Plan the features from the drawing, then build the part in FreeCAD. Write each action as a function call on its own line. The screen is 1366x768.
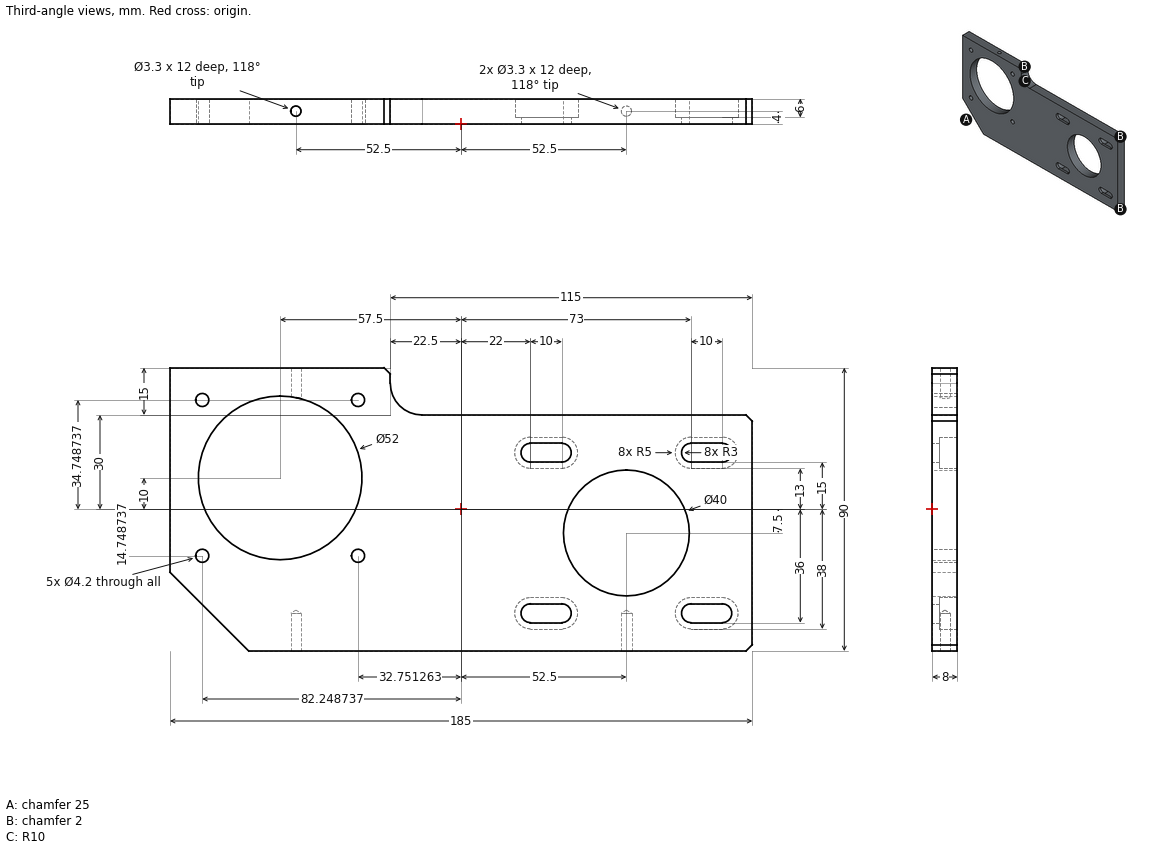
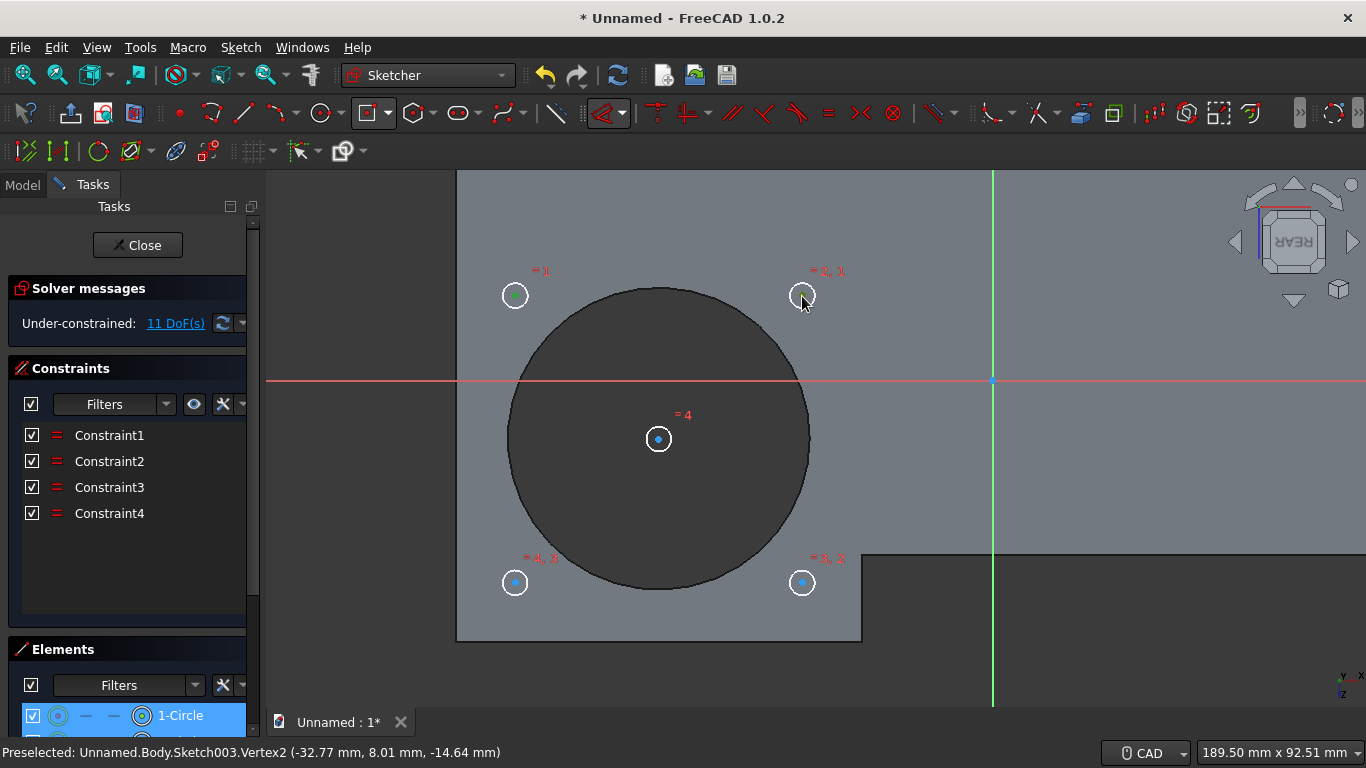
key(h)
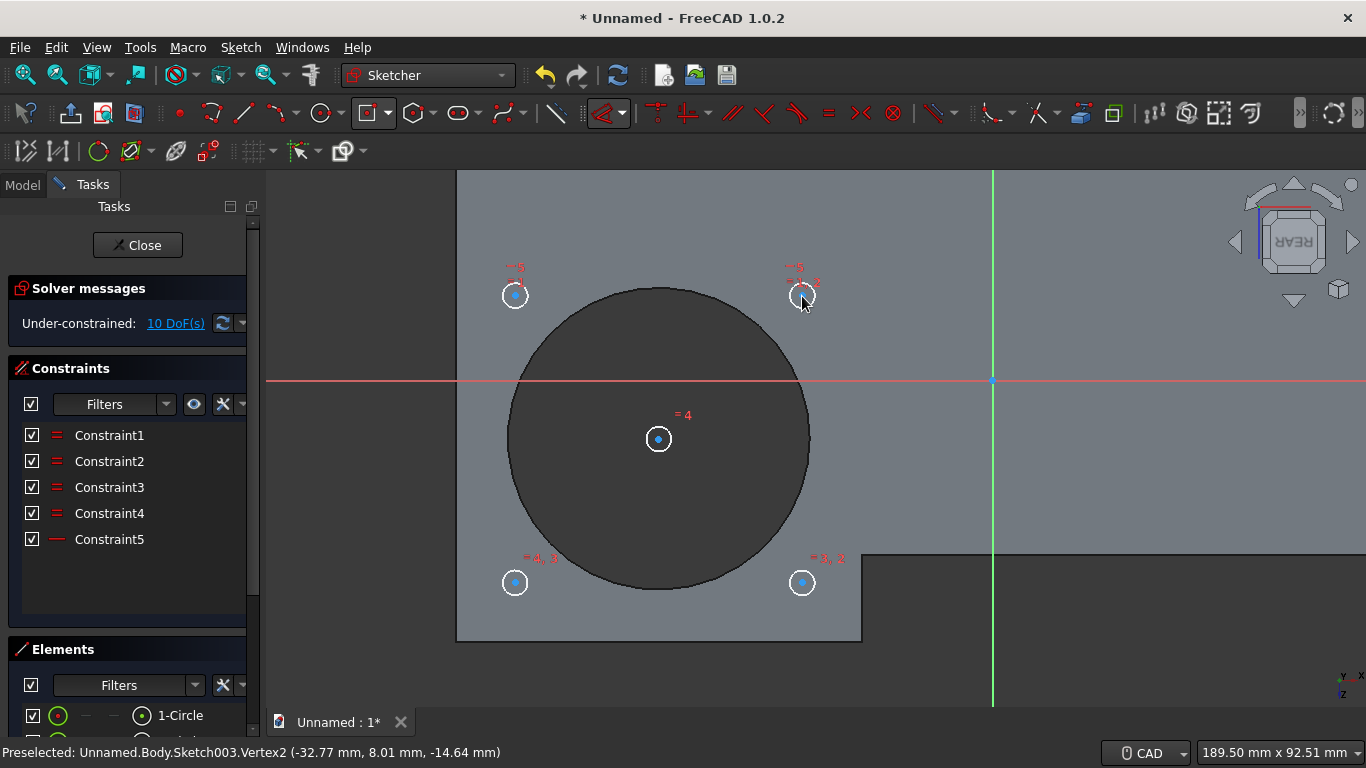
click(802, 296)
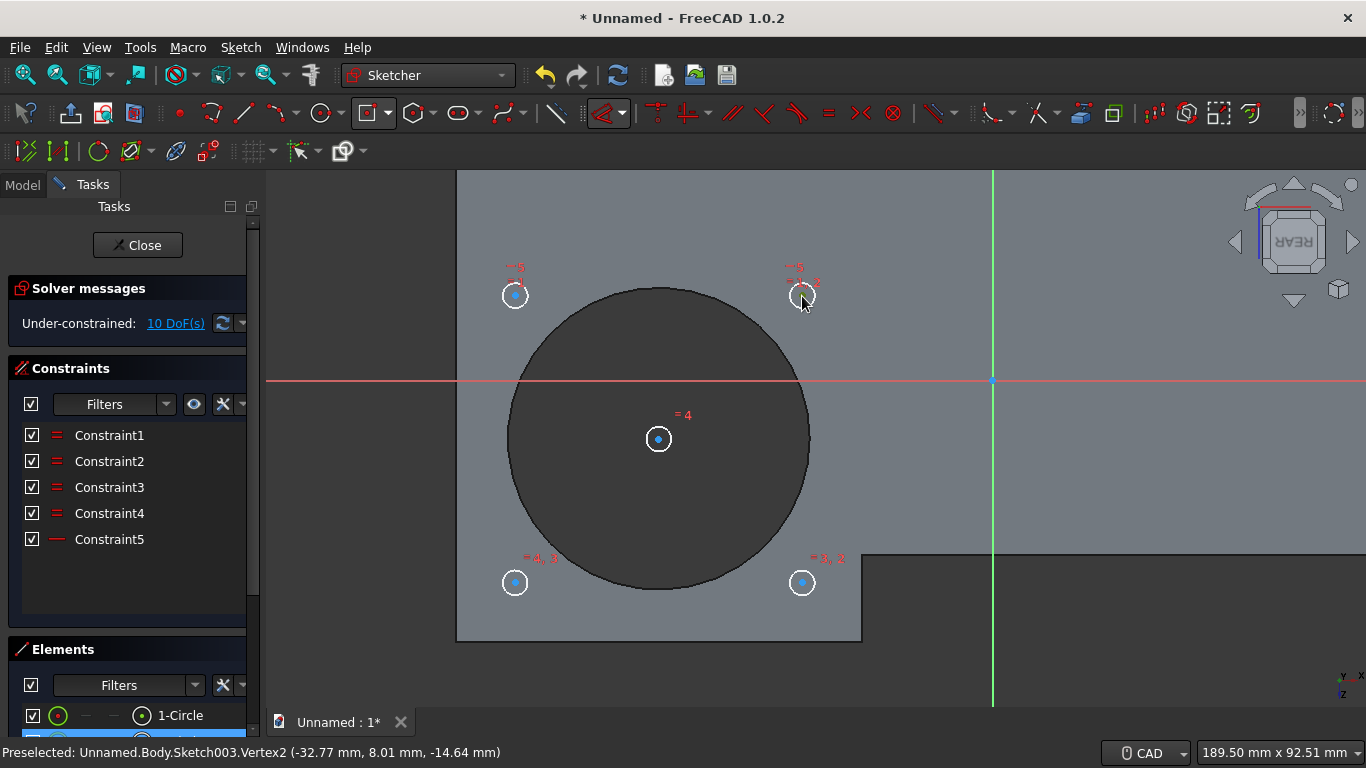
click(802, 583)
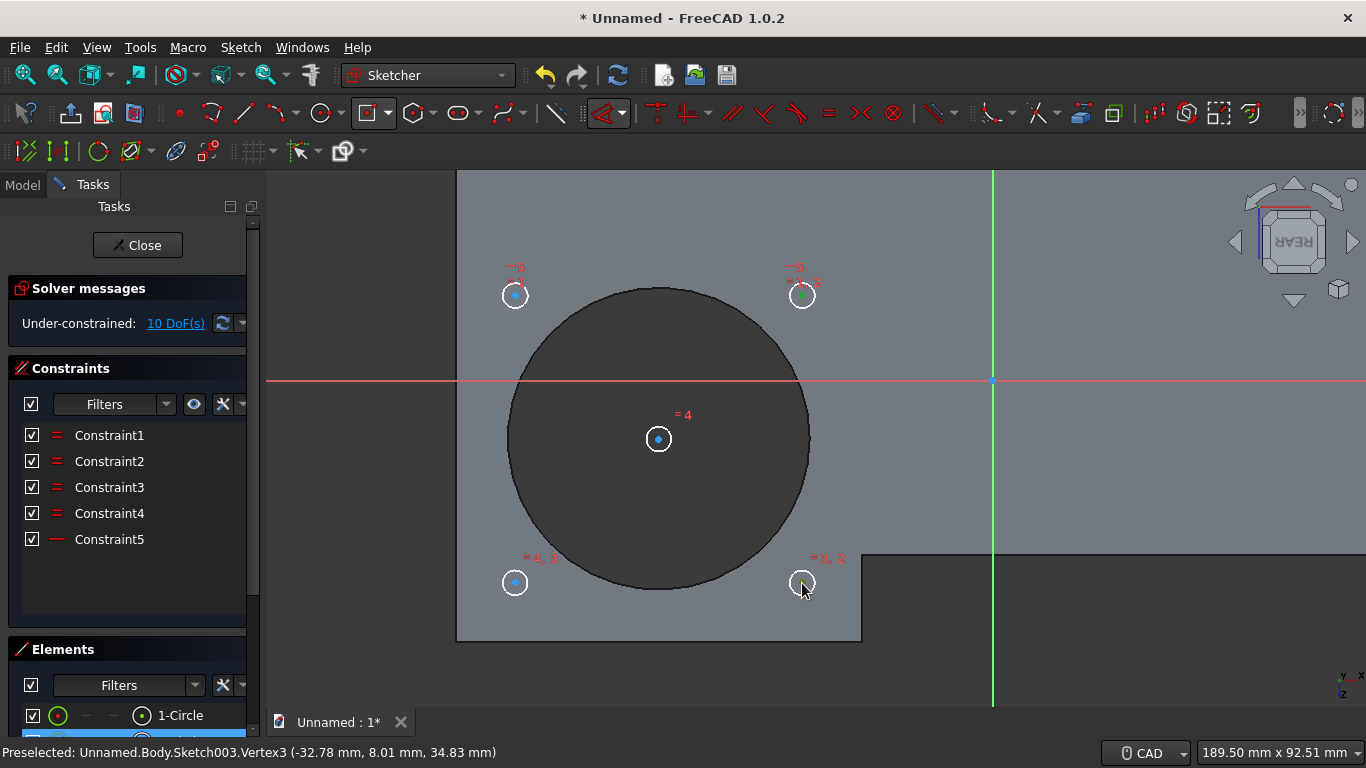
key(v)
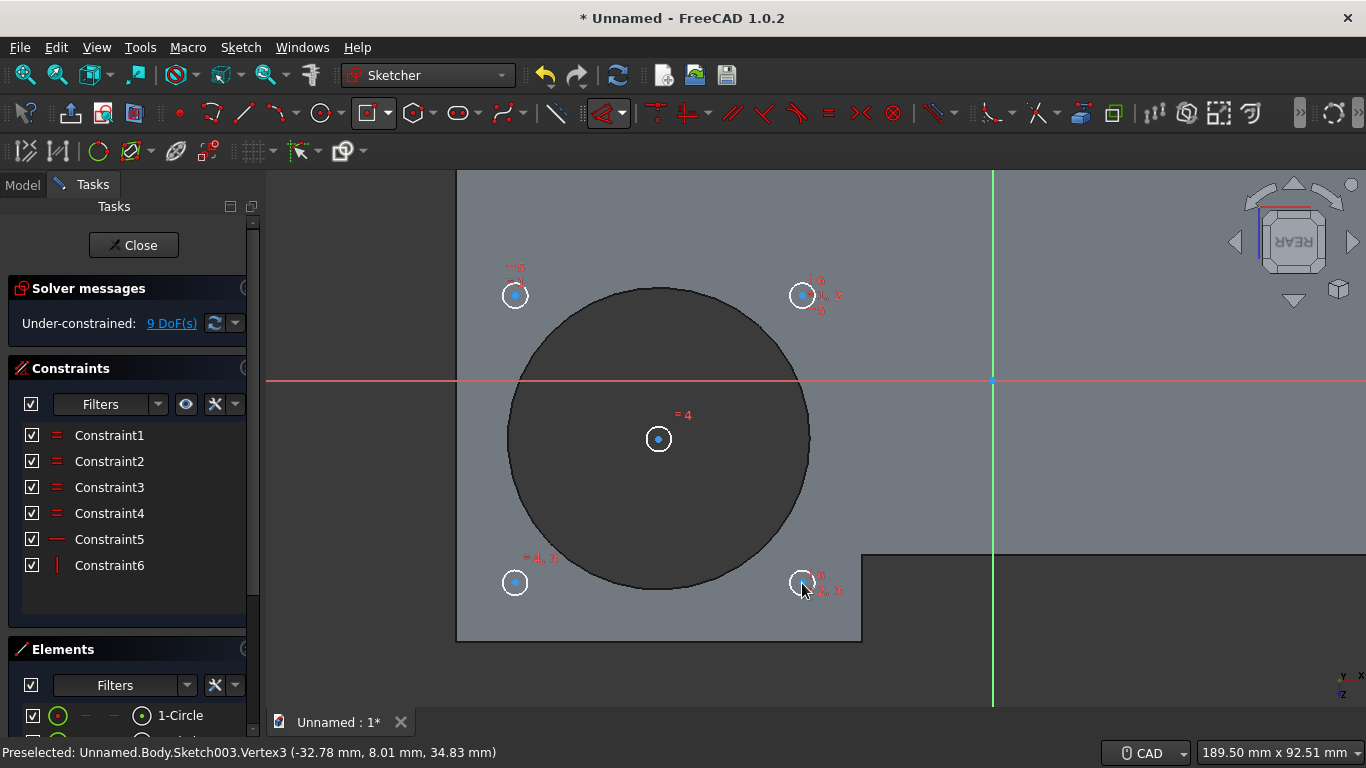
click(515, 296)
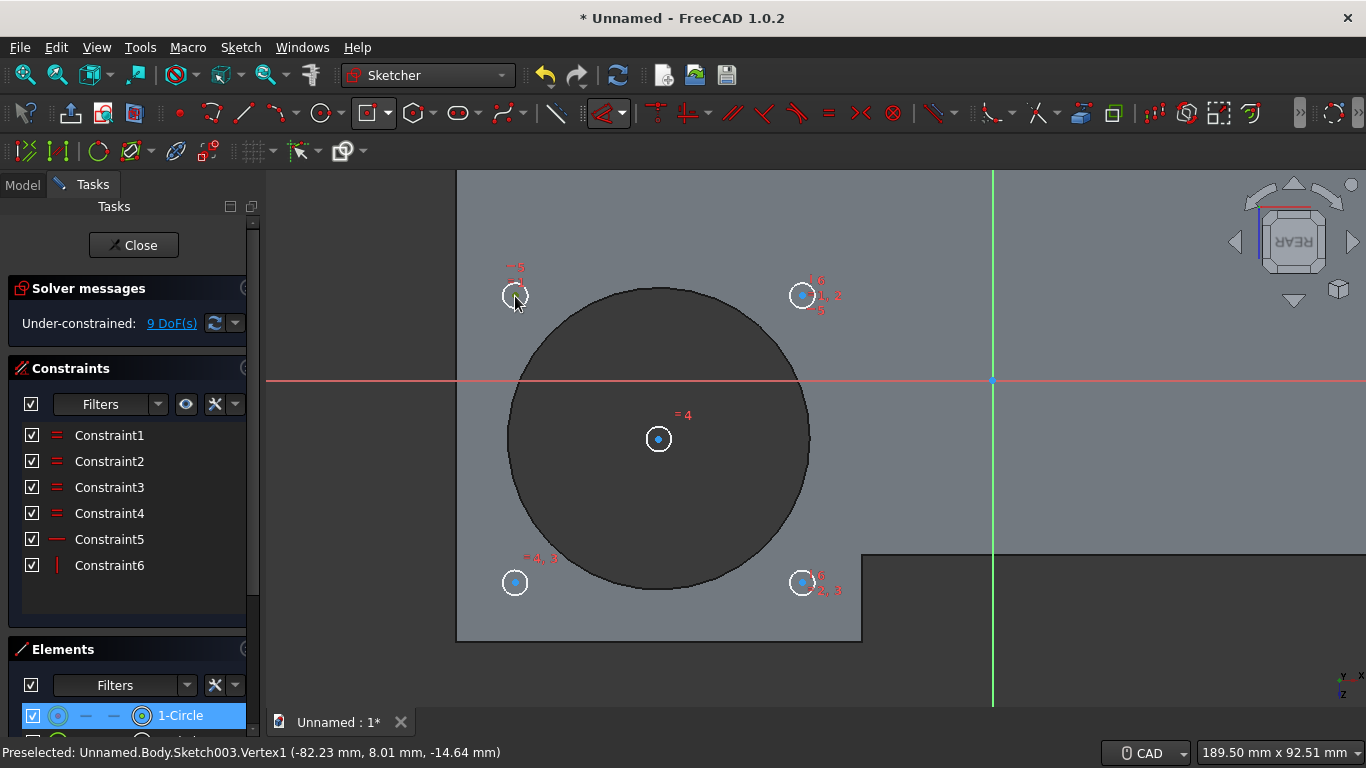
click(515, 583)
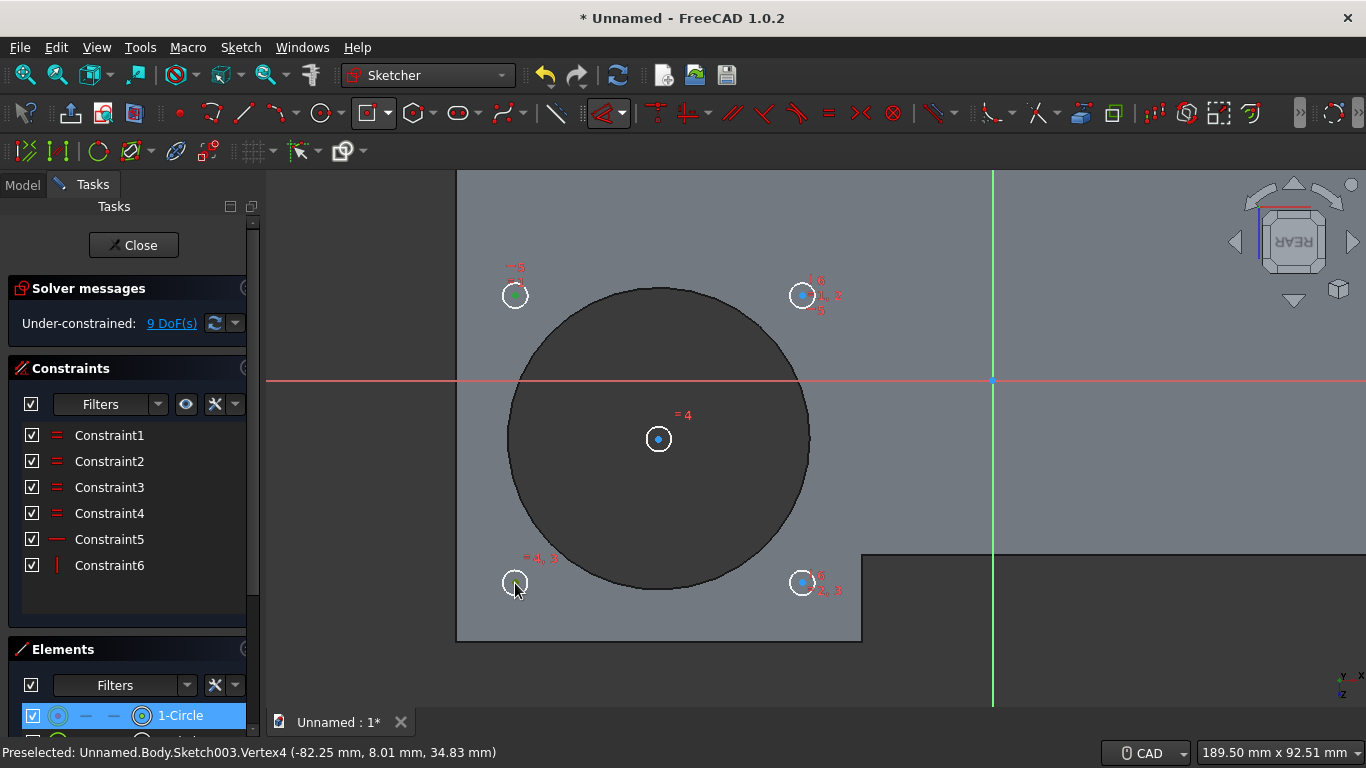
key(v)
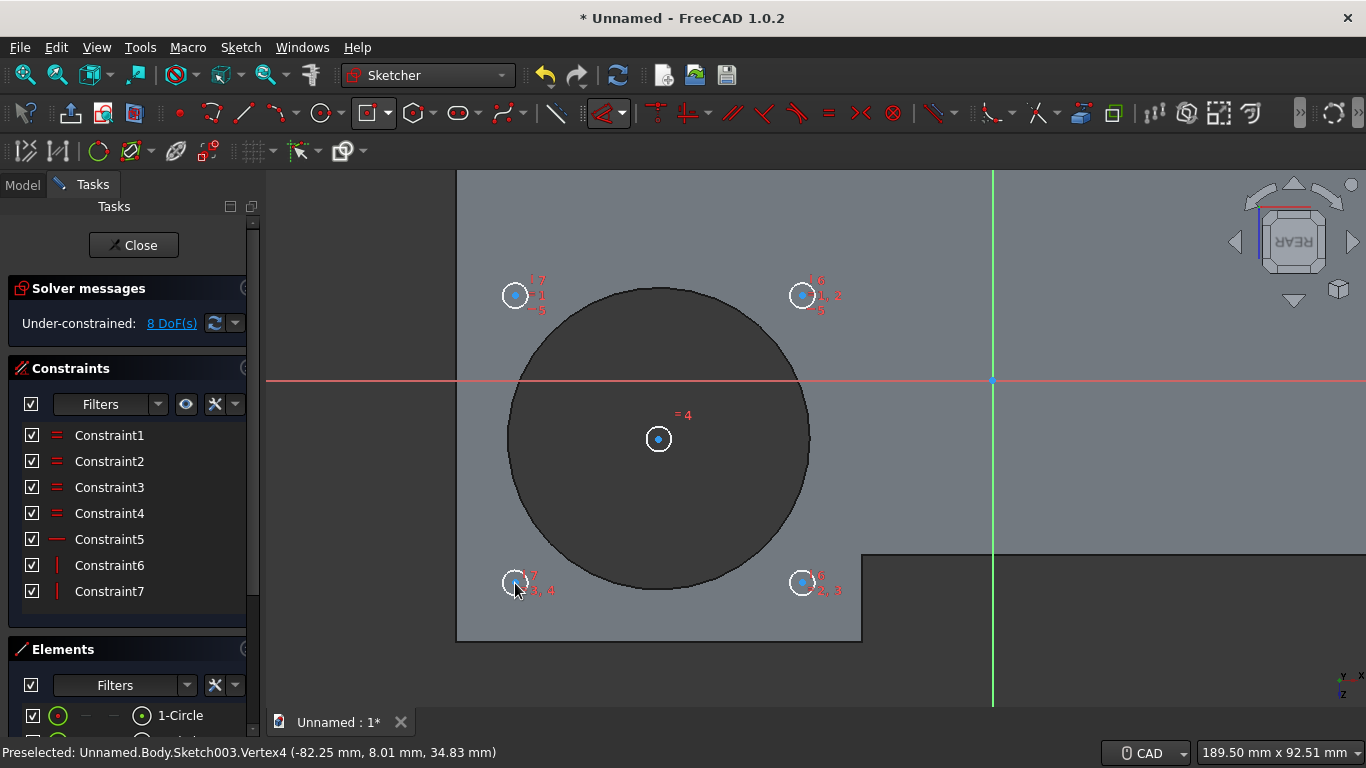
click(802, 583)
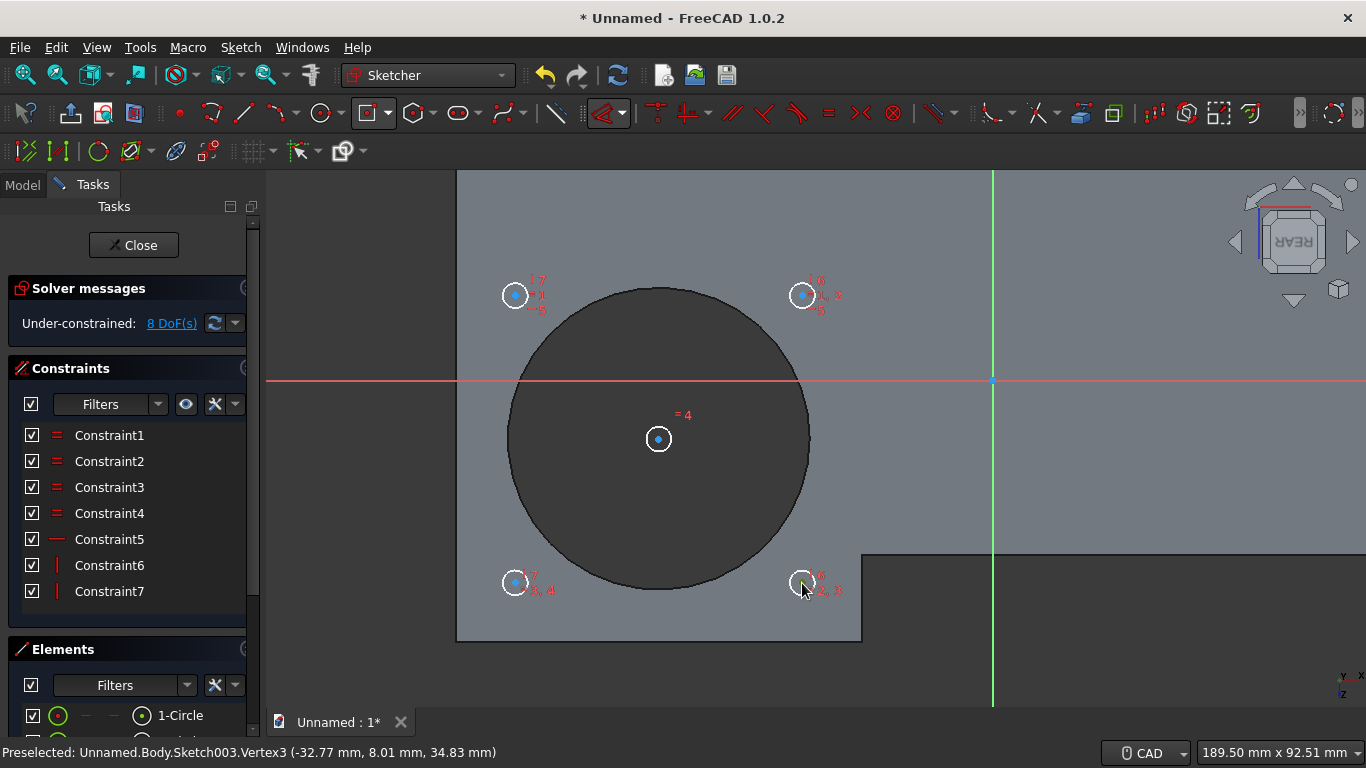
click(515, 583)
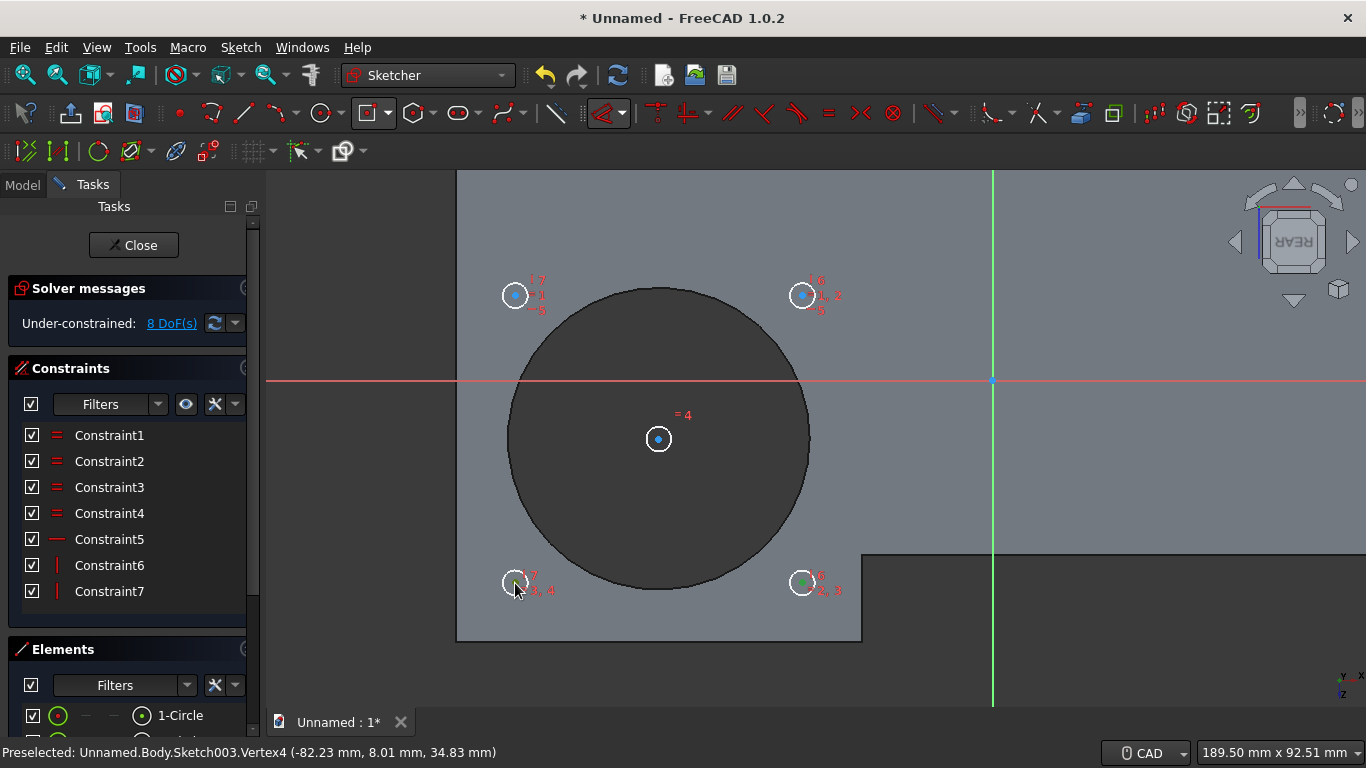
key(h)